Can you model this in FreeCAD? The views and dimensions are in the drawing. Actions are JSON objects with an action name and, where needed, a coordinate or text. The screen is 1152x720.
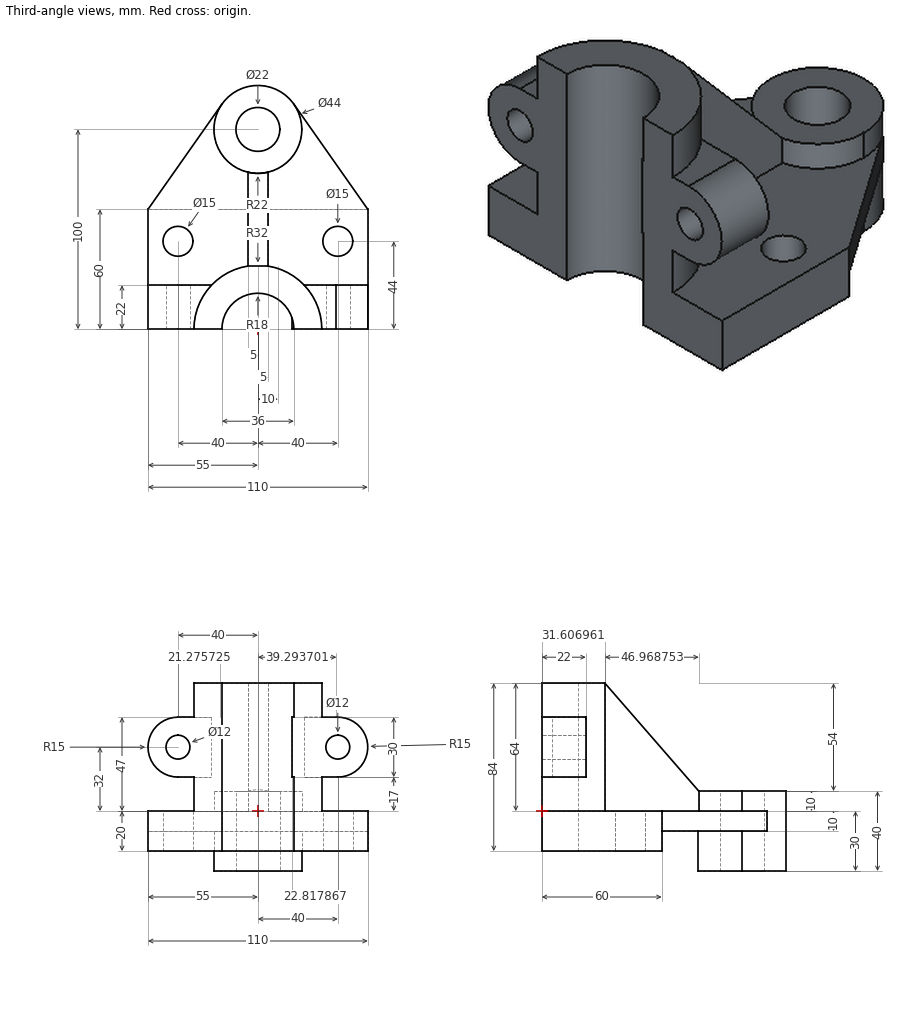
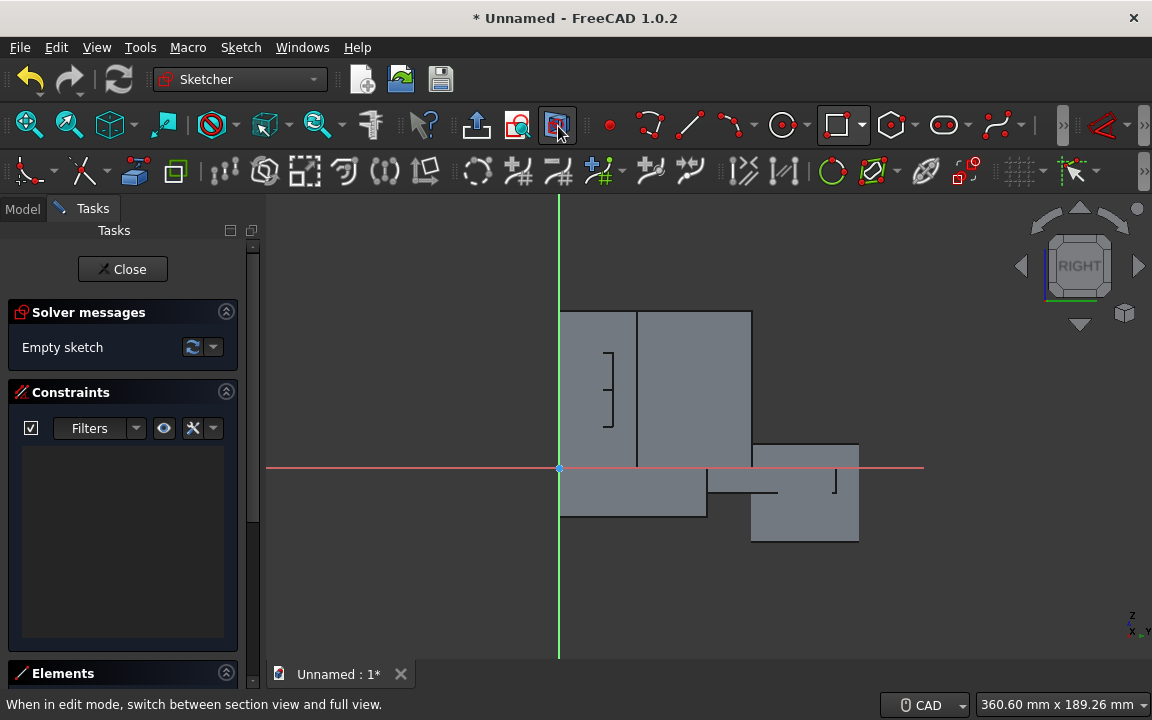
{"action": "scroll", "coordinate": [674, 345], "scroll_direction": "up", "scroll_amount": 3}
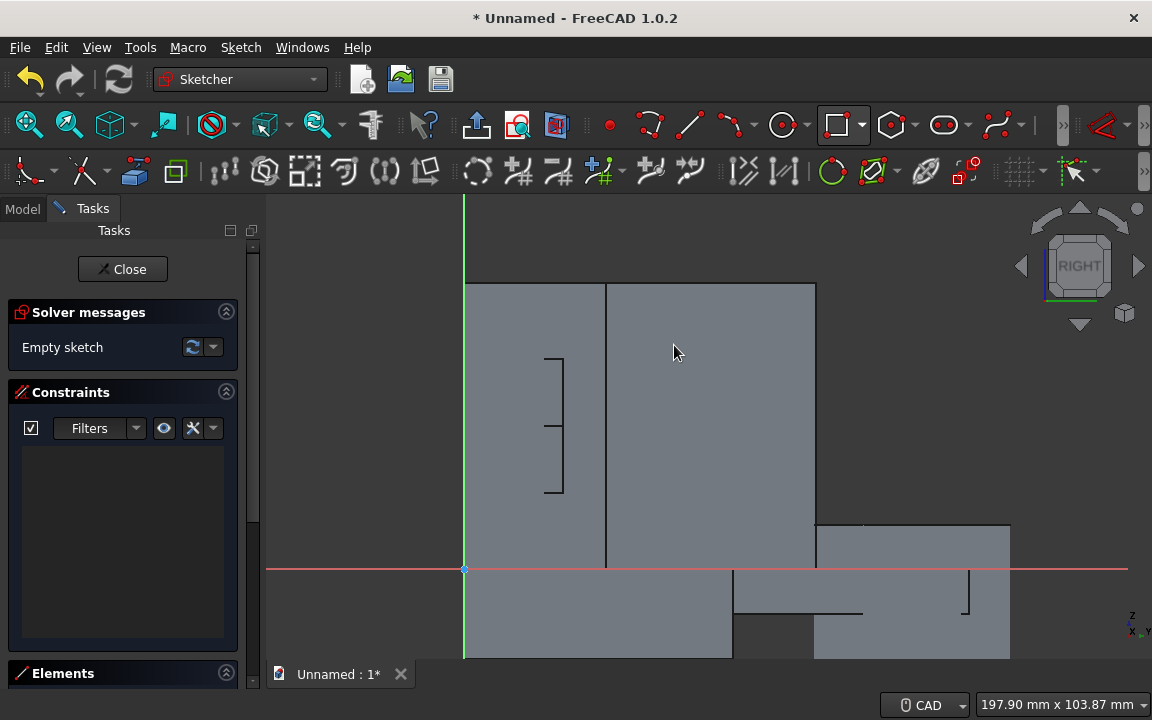
{"action": "left_click", "coordinate": [650, 126]}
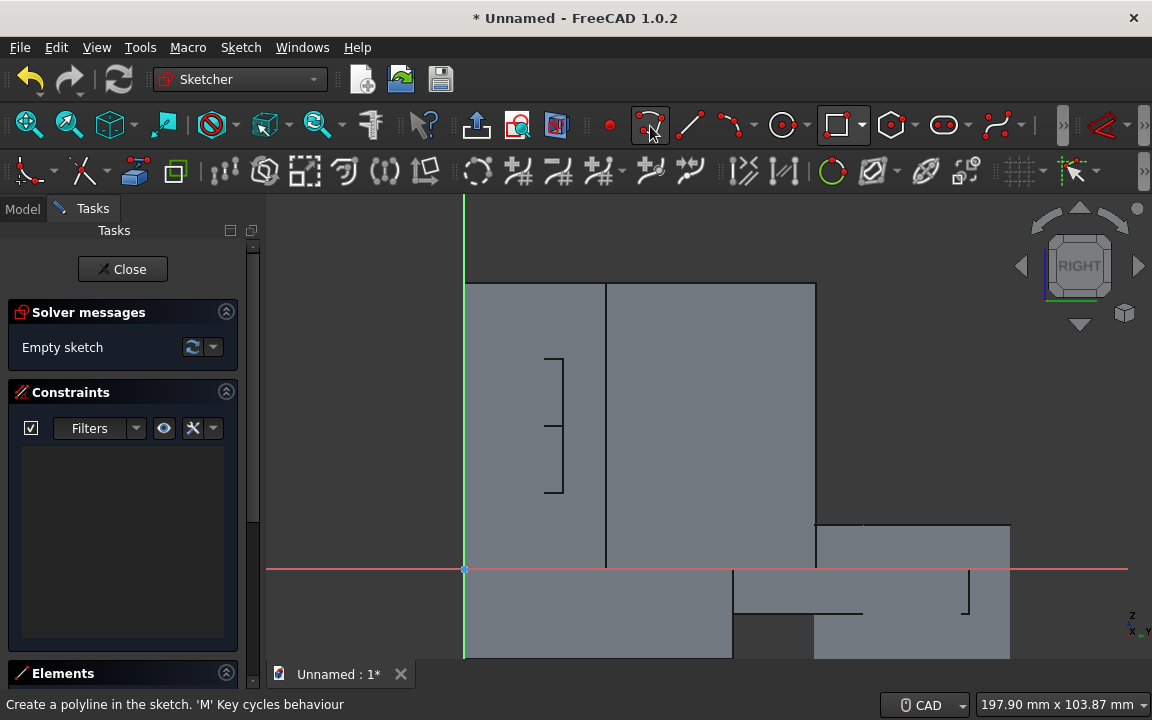
{"action": "left_click", "coordinate": [606, 283]}
{"action": "left_click", "coordinate": [816, 525]}
{"action": "left_click", "coordinate": [816, 283]}
{"action": "left_click", "coordinate": [606, 284]}
{"action": "key", "text": "Escape"}
{"action": "key", "text": "Escape"}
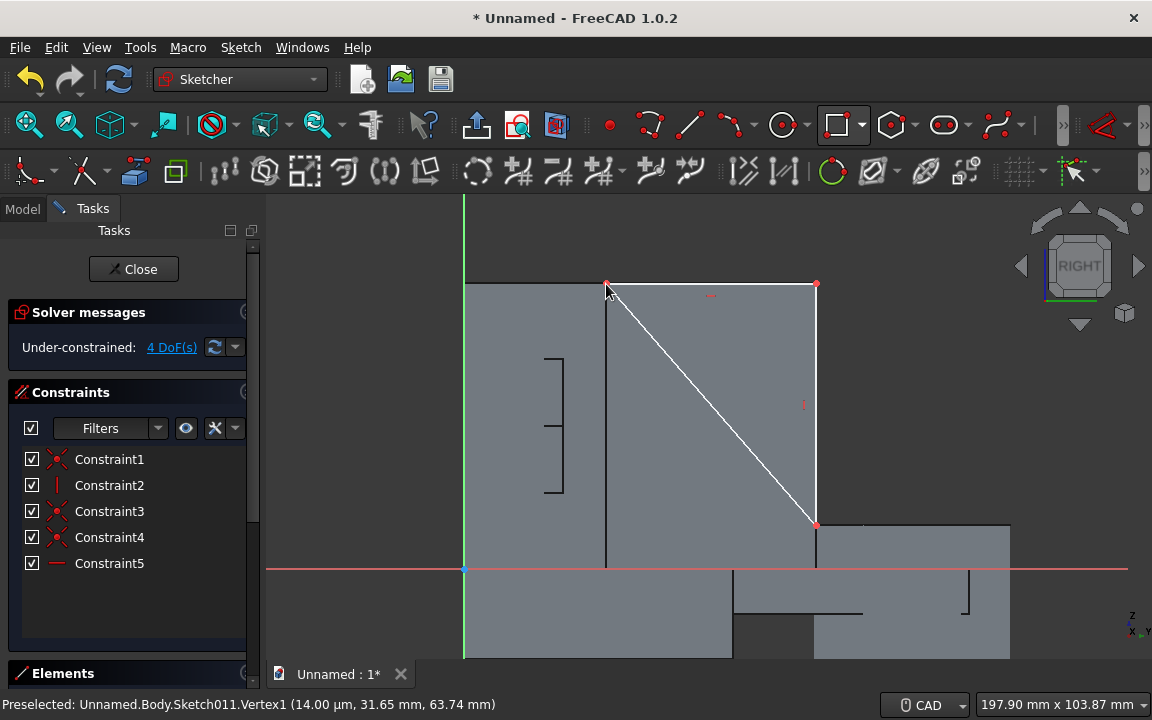
{"action": "left_click", "coordinate": [1102, 126]}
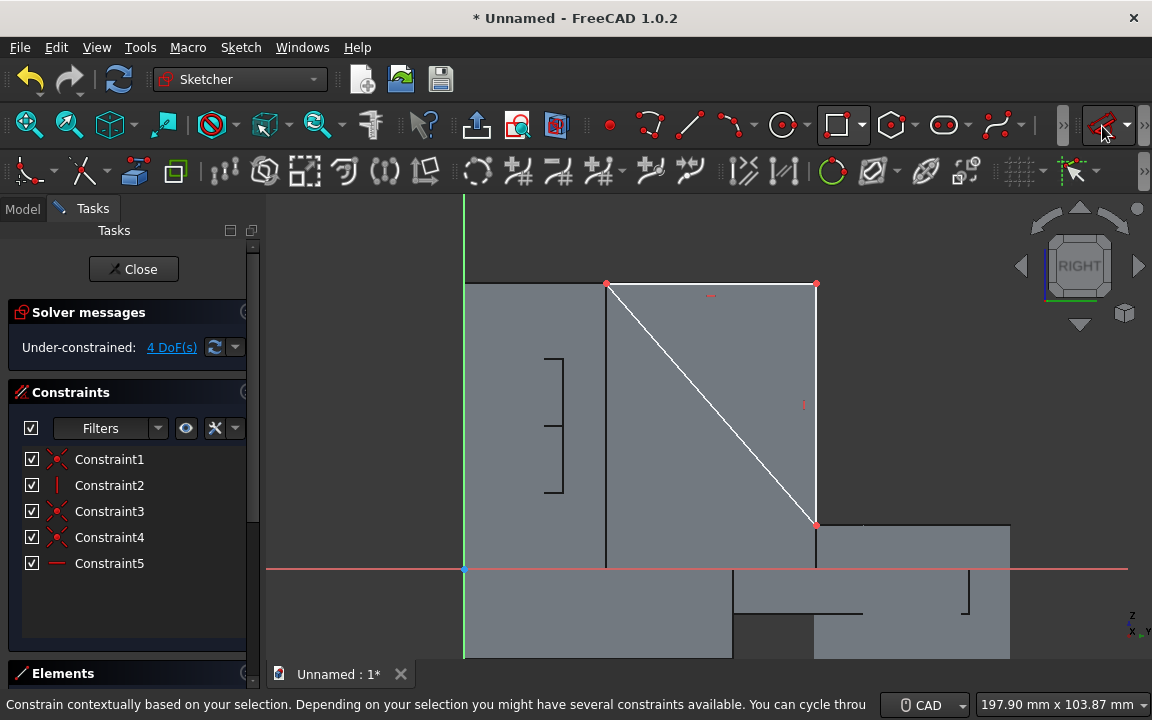
{"action": "left_click", "coordinate": [816, 453]}
{"action": "left_click", "coordinate": [850, 405]}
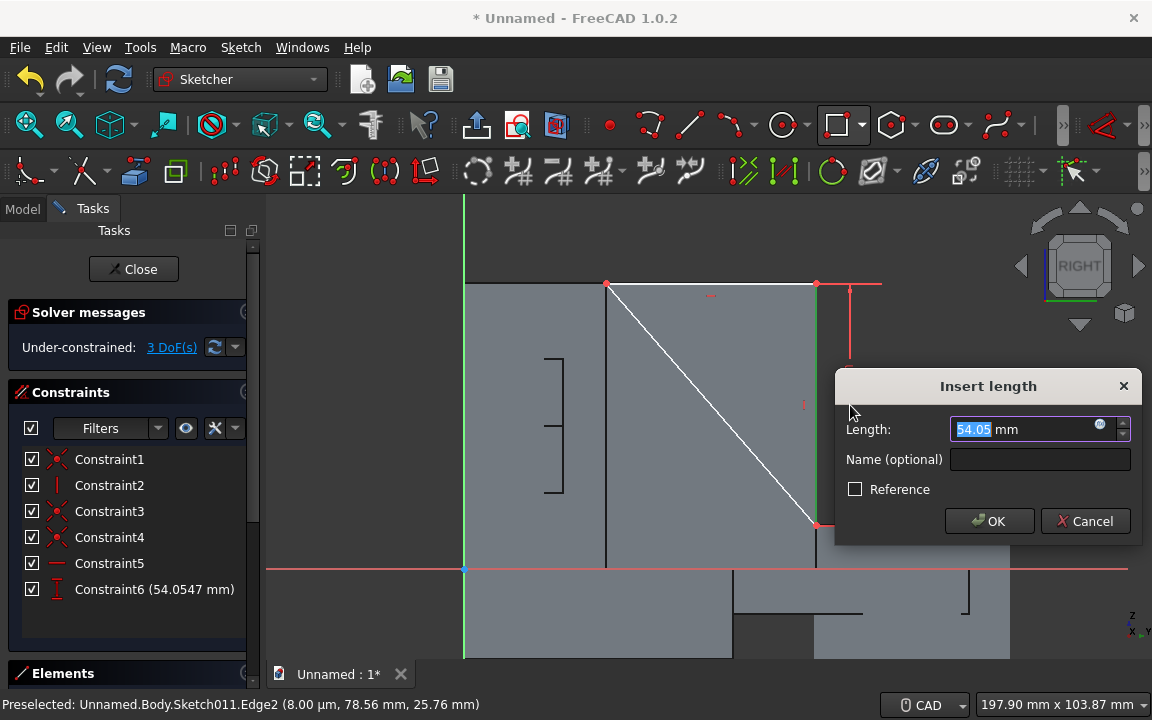
{"action": "type", "text": "54"}
{"action": "key", "text": "Return"}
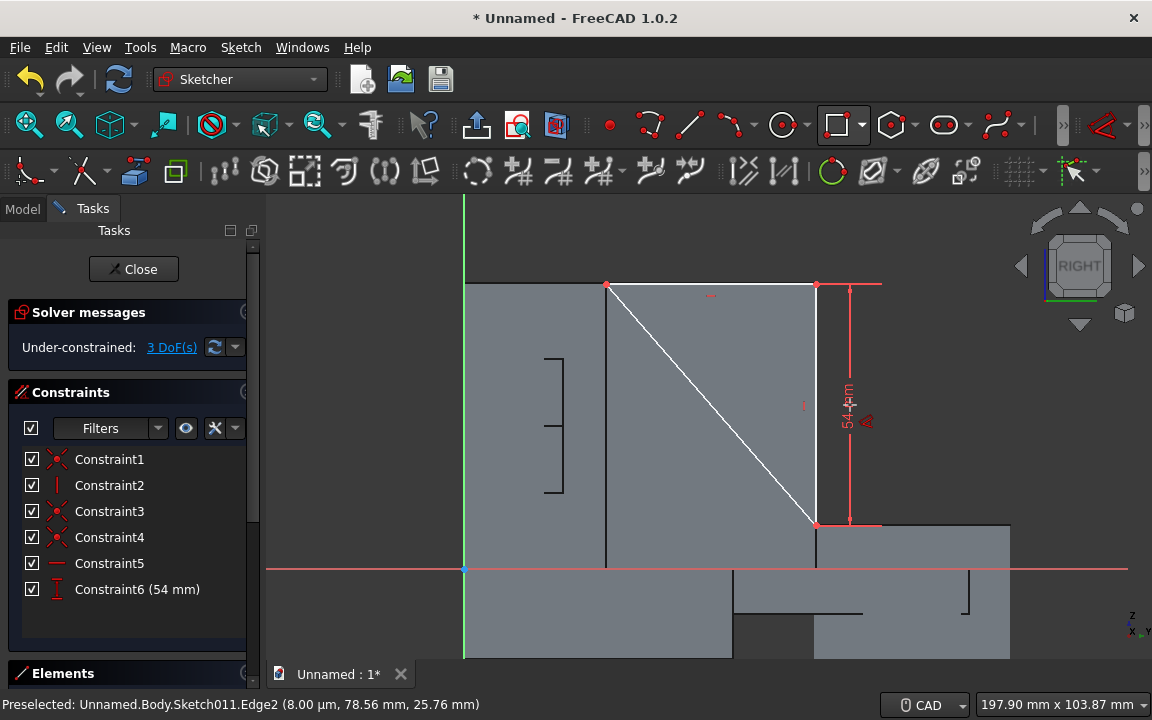
{"action": "left_click", "coordinate": [606, 284]}
{"action": "left_click", "coordinate": [430, 427]}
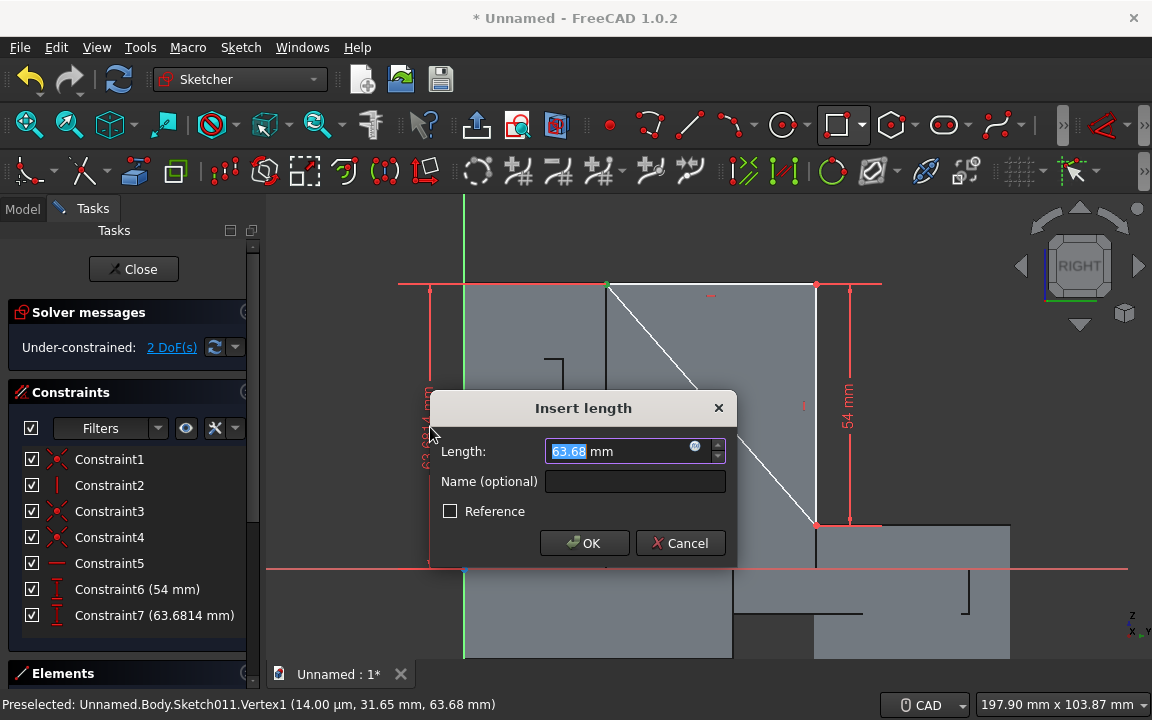
{"action": "type", "text": "64"}
{"action": "key", "text": "Return"}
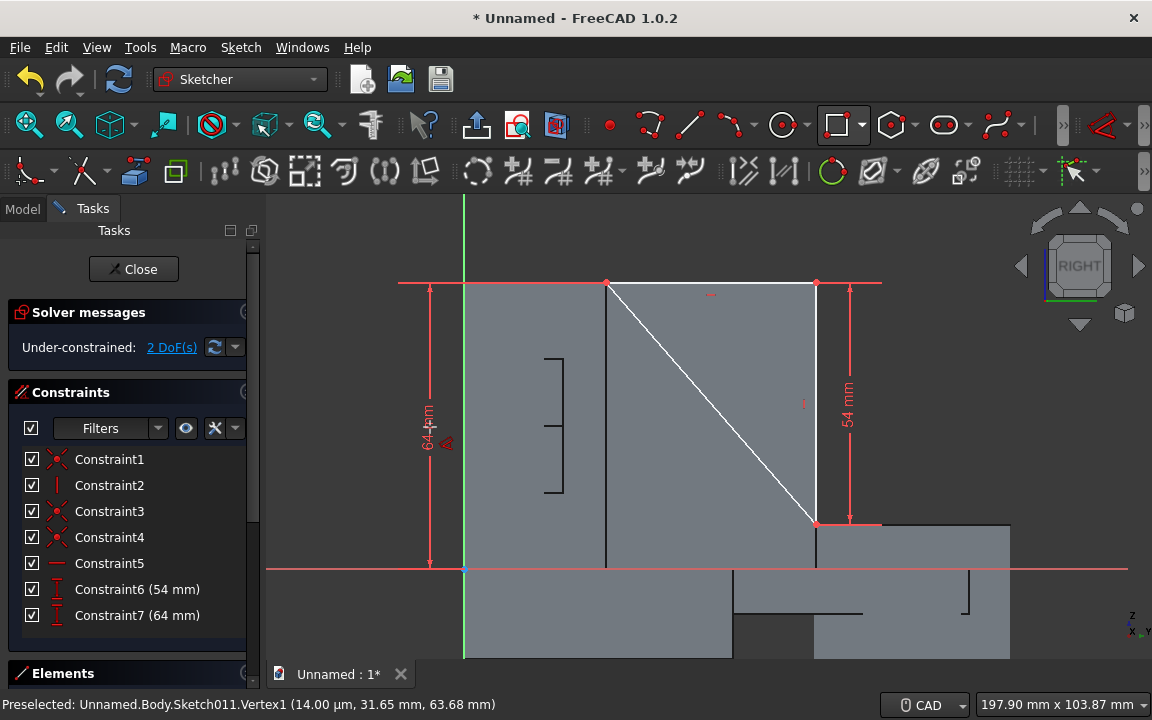
{"action": "left_click", "coordinate": [753, 283]}
{"action": "left_click", "coordinate": [711, 249]}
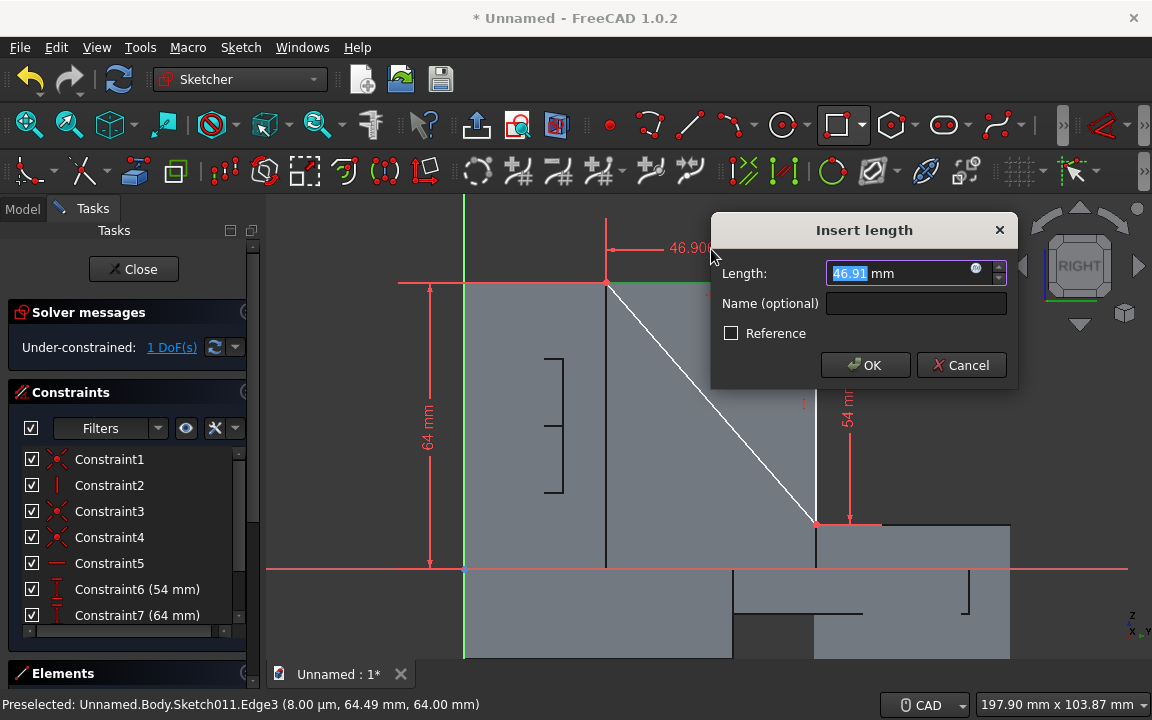
{"action": "type", "text": "46.968753"}
{"action": "key", "text": "Return"}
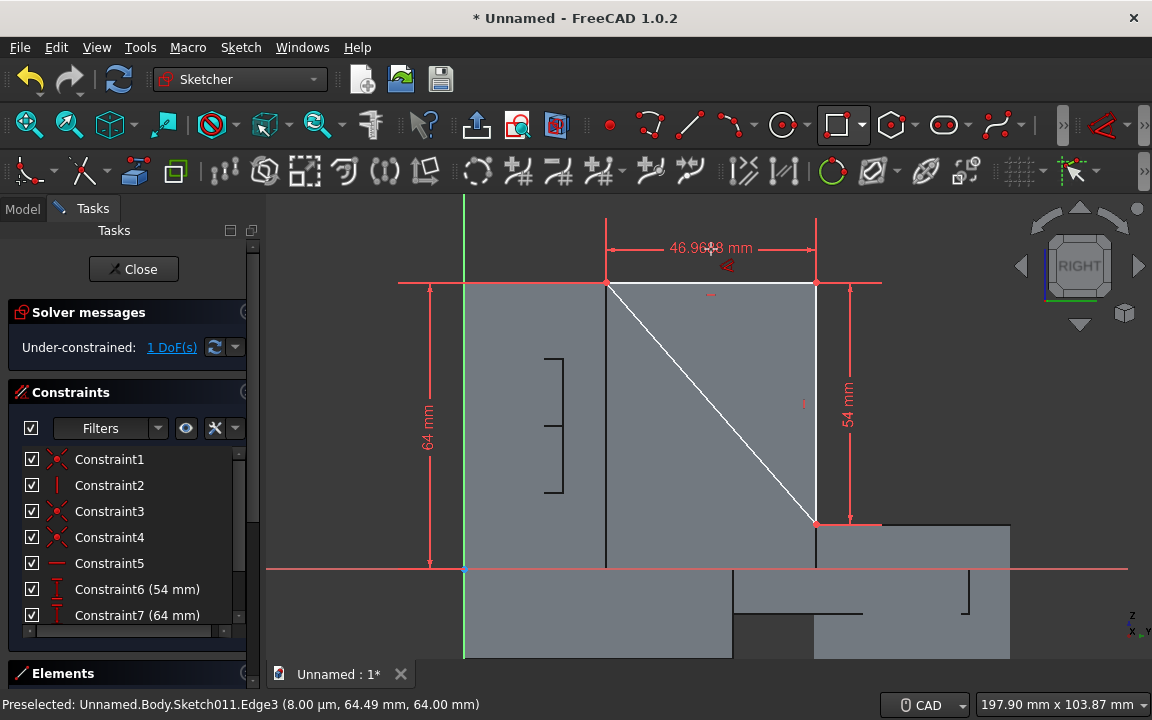
{"action": "left_click", "coordinate": [606, 283]}
{"action": "left_click", "coordinate": [535, 603]}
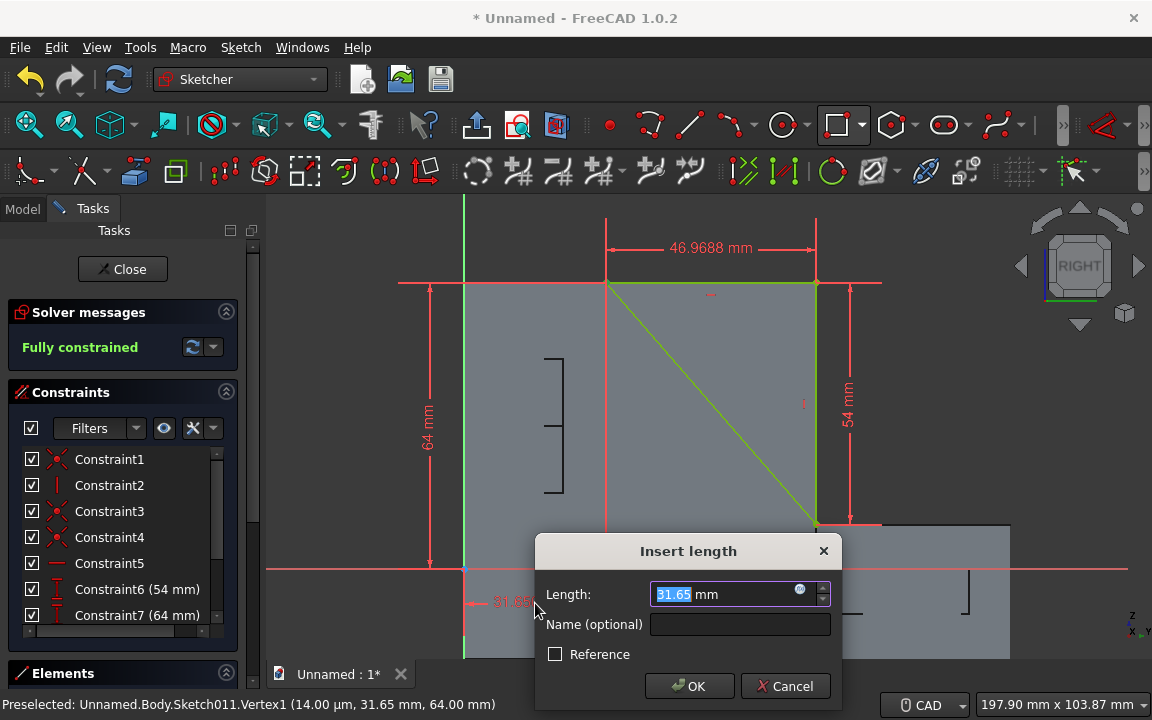
{"action": "type", "text": "31.606961"}
{"action": "key", "text": "Return"}
{"action": "key", "text": "Escape"}